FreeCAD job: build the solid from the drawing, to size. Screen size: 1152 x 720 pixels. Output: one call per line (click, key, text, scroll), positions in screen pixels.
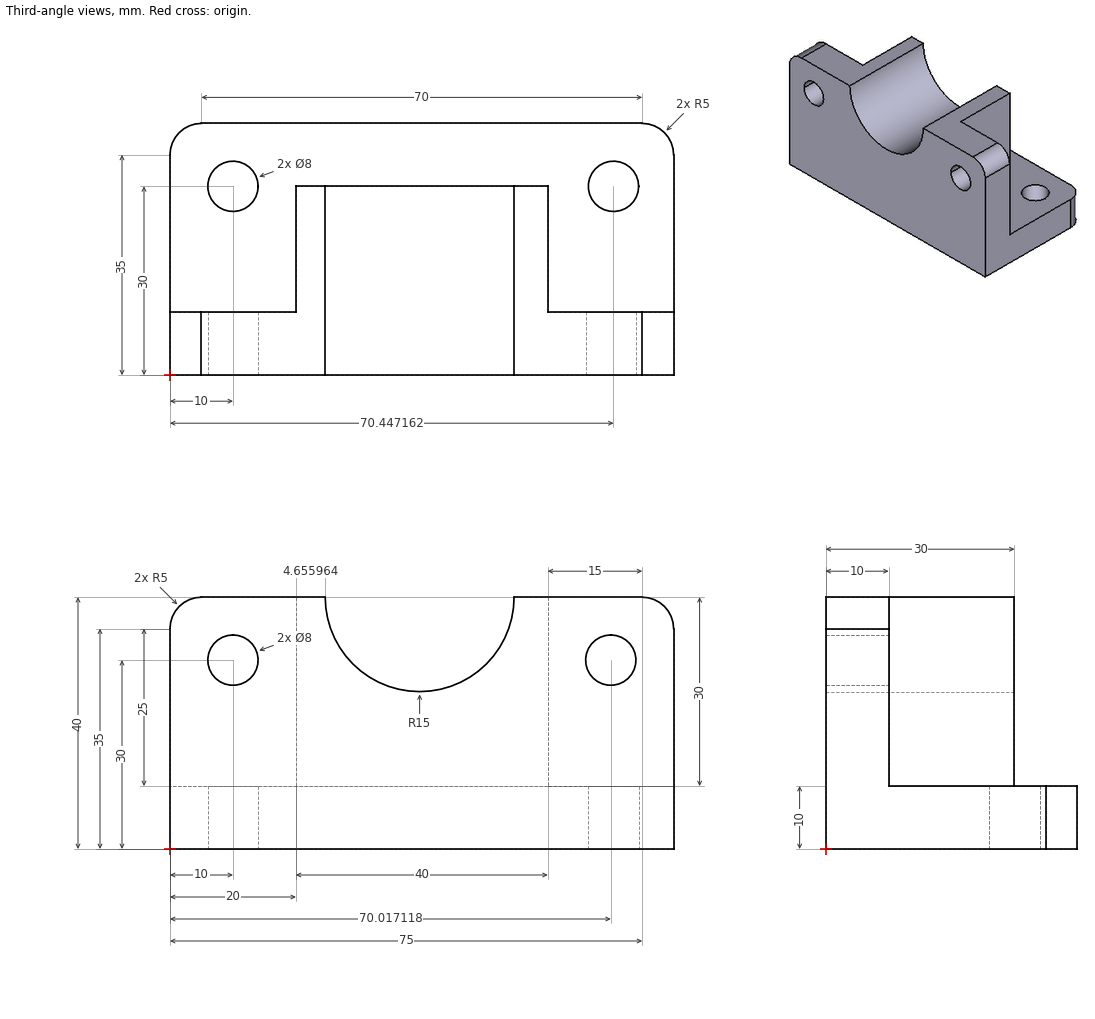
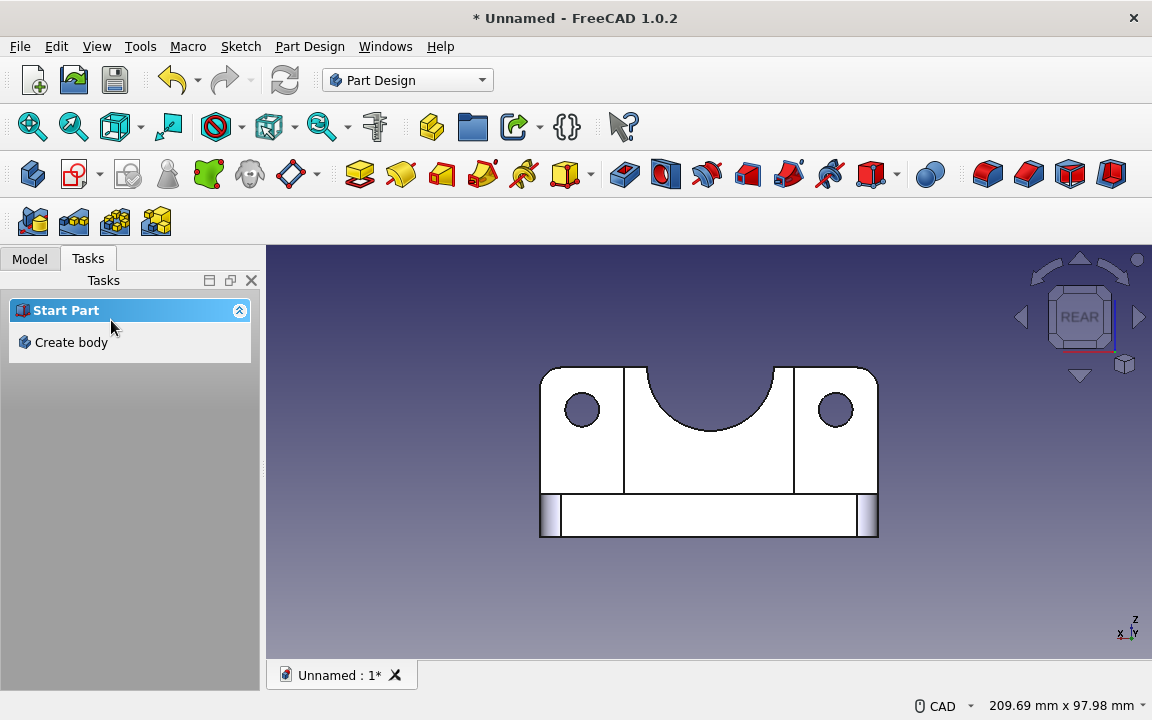
key(0)